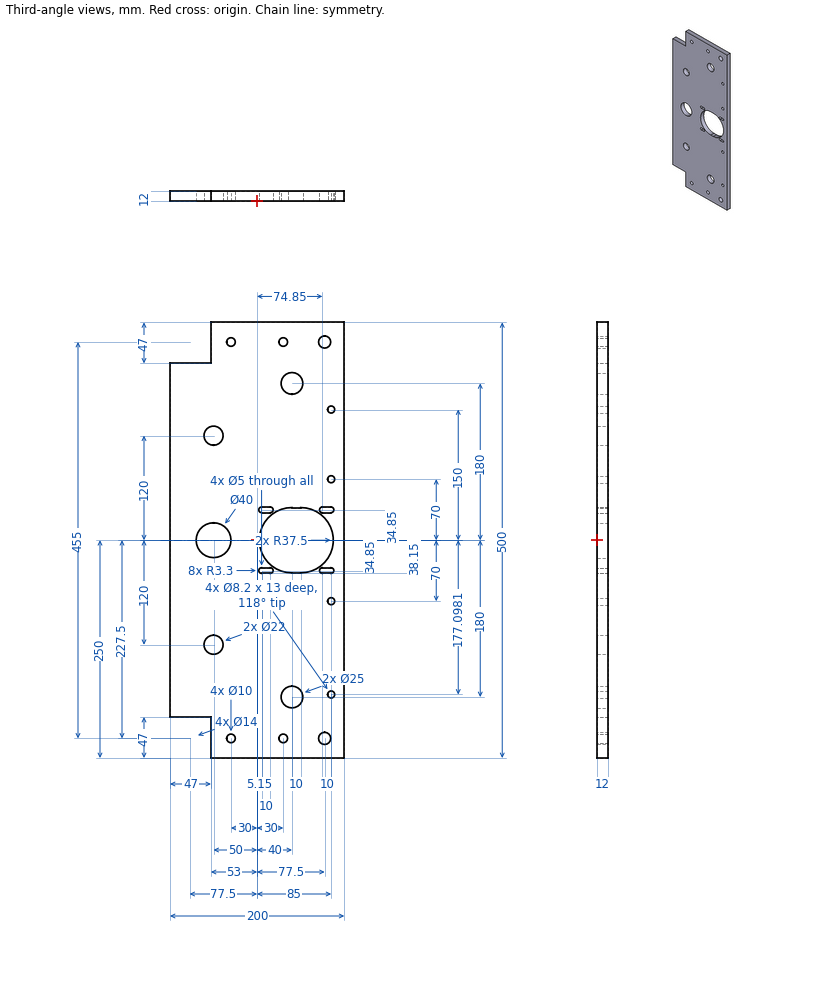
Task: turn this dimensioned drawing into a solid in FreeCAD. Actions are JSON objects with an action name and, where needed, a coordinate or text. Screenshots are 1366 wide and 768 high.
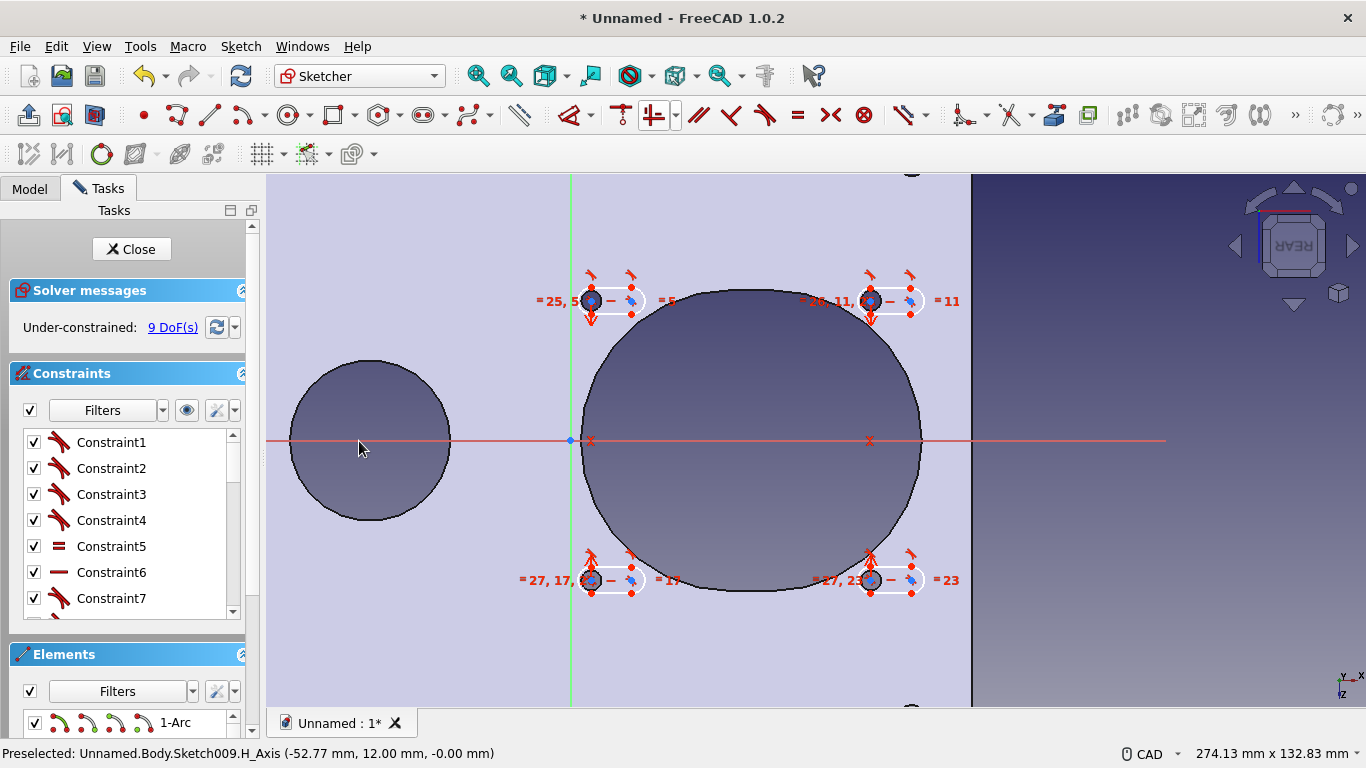
{"action": "scroll", "coordinate": [581, 293], "scroll_direction": "up", "scroll_amount": 6}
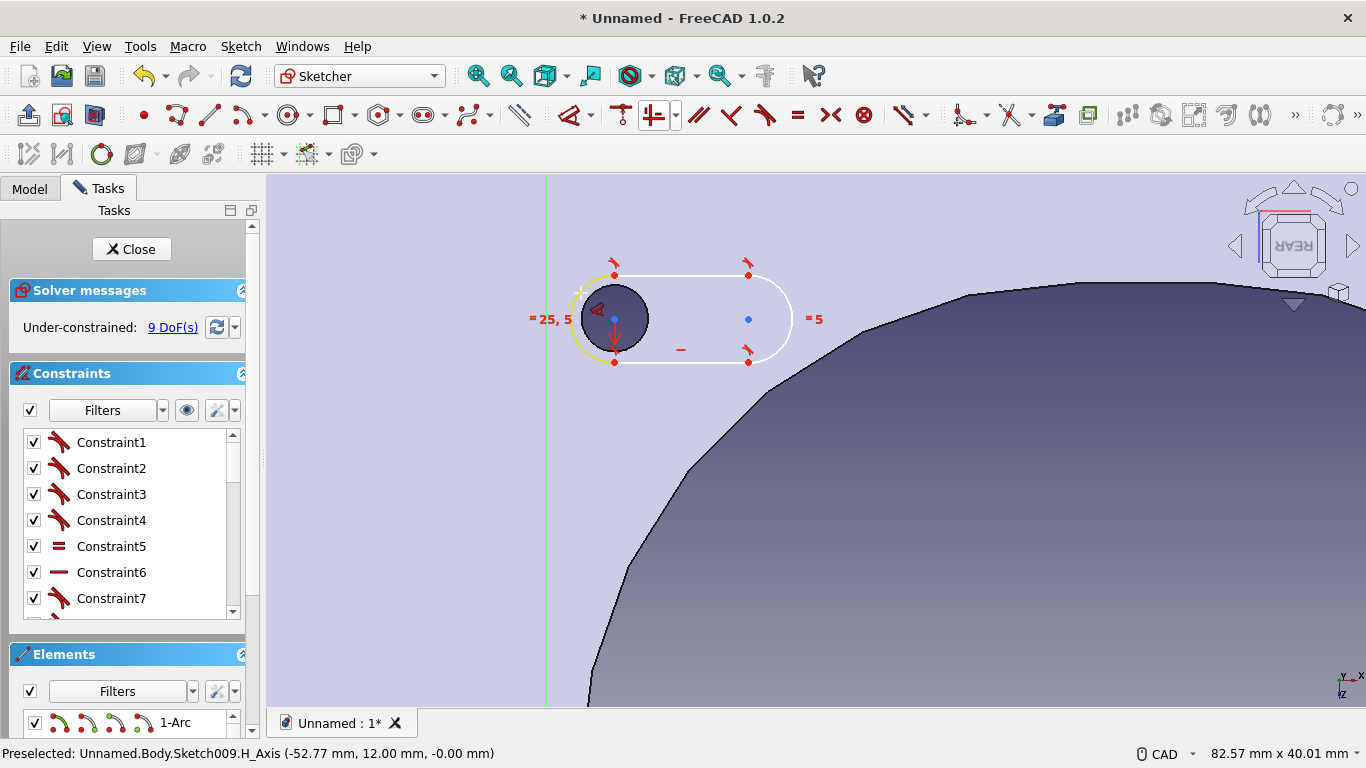
{"action": "left_click", "coordinate": [579, 294]}
{"action": "left_click", "coordinate": [581, 251]}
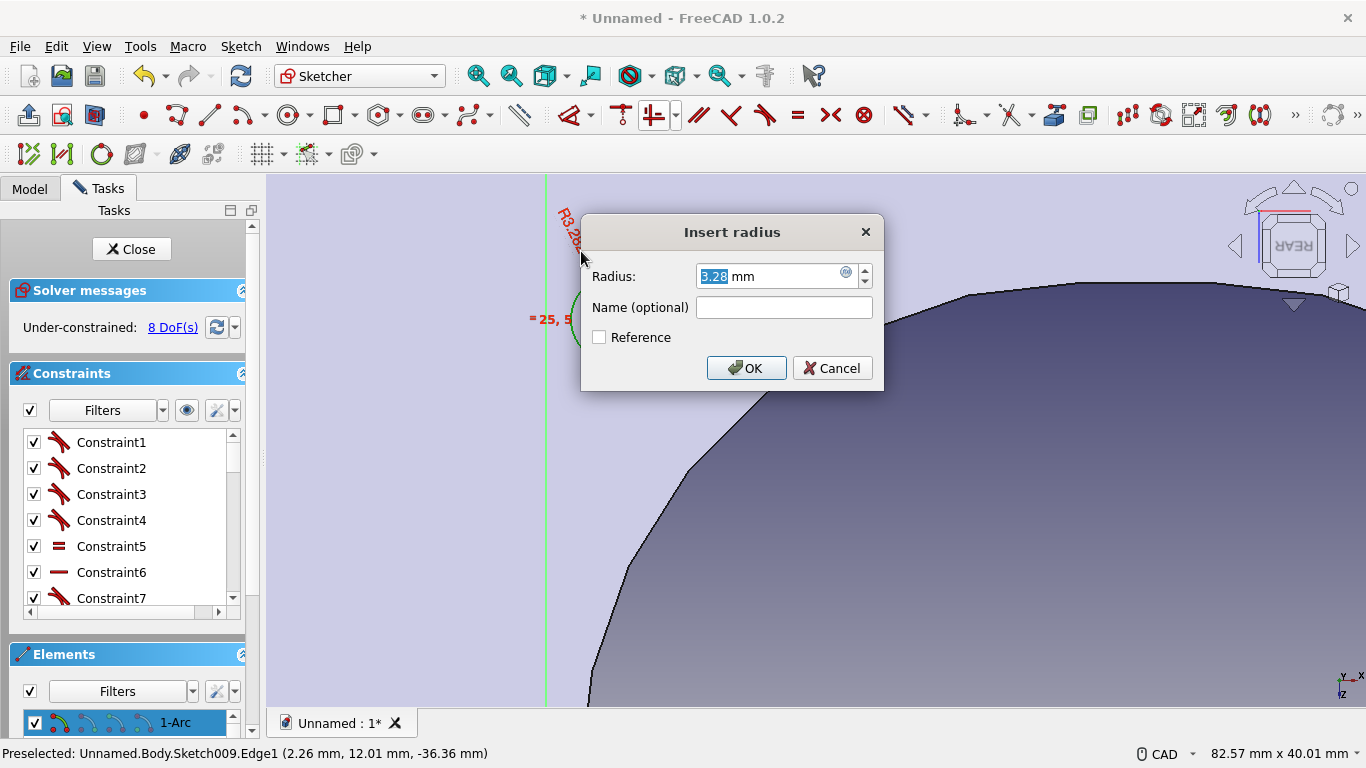
{"action": "type", "text": "3.3"}
{"action": "key", "text": "Return"}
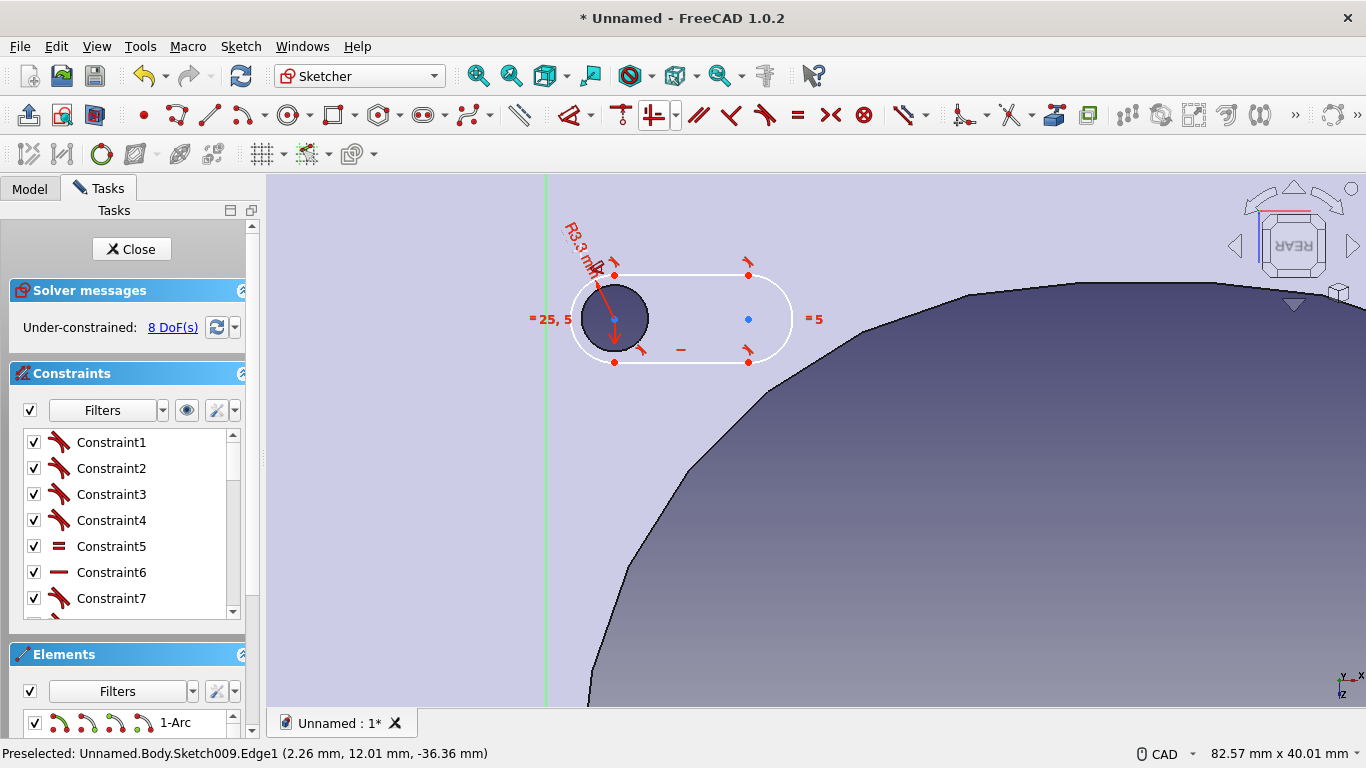
{"action": "left_click", "coordinate": [655, 275]}
{"action": "left_click", "coordinate": [682, 241]}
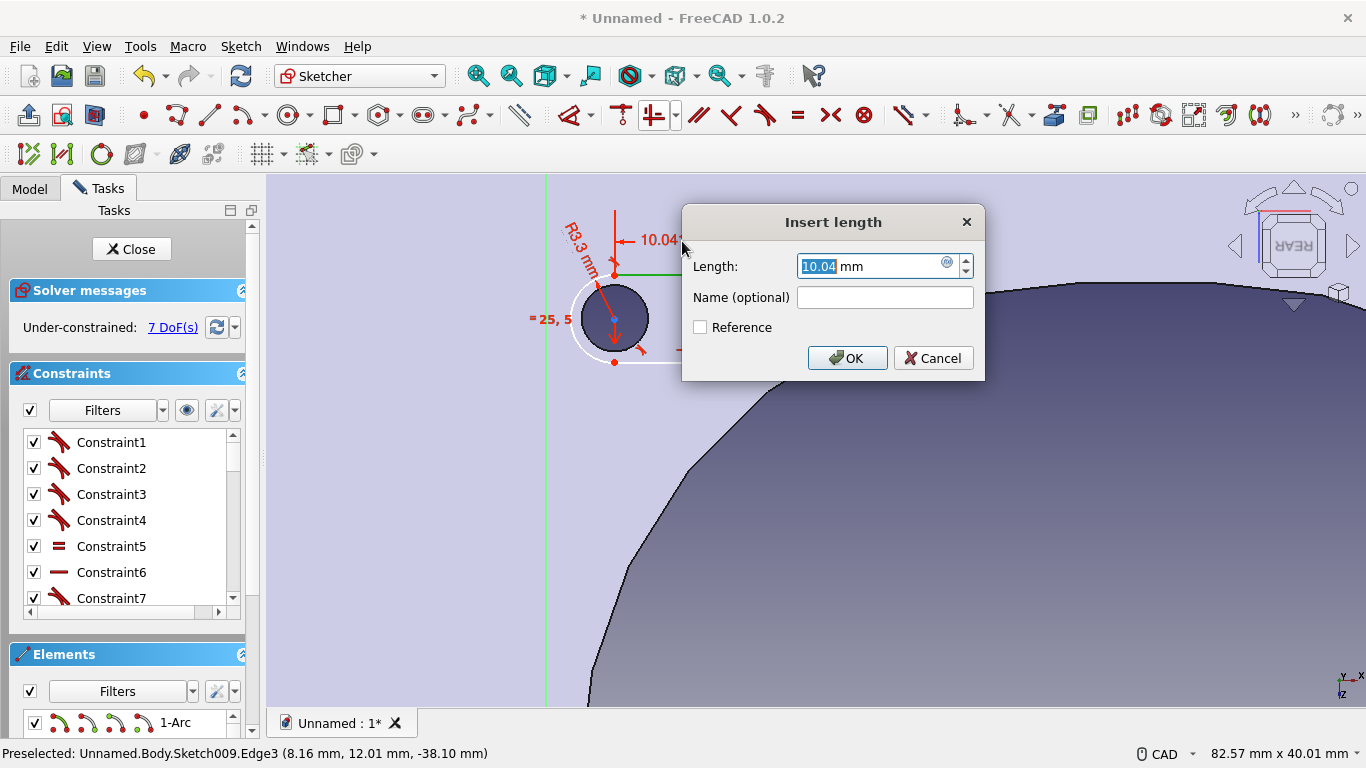
{"action": "type", "text": "10"}
{"action": "key", "text": "Return"}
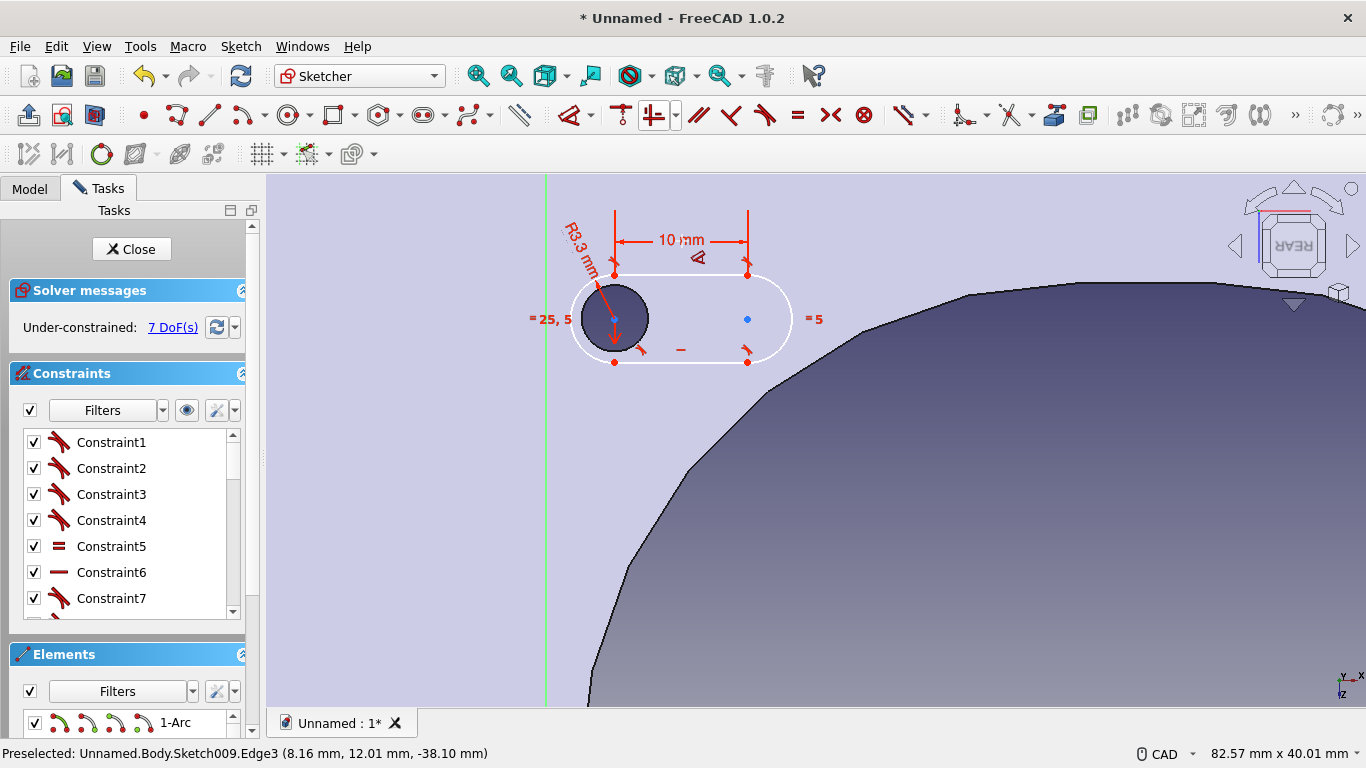
{"action": "scroll", "coordinate": [581, 293], "scroll_direction": "down", "scroll_amount": 6}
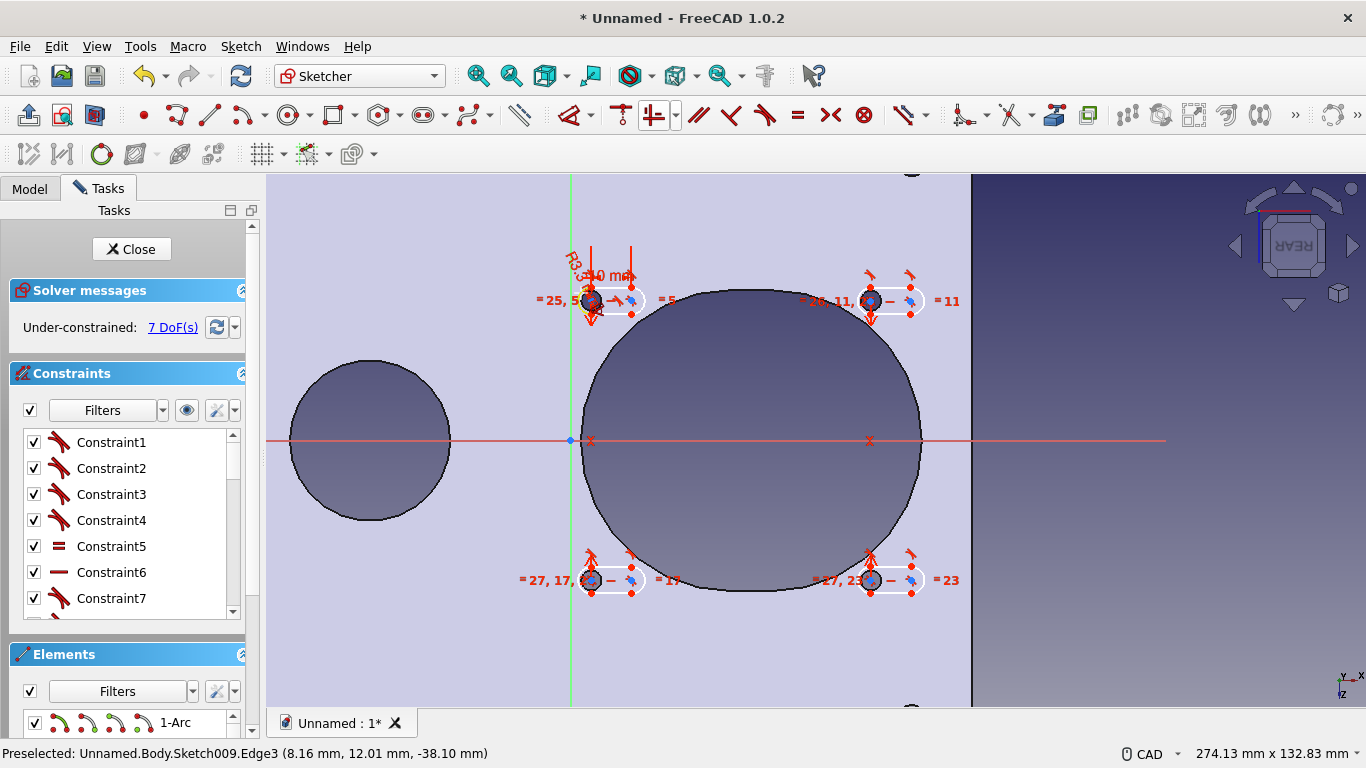
{"action": "left_click", "coordinate": [883, 288]}
{"action": "left_click", "coordinate": [891, 254]}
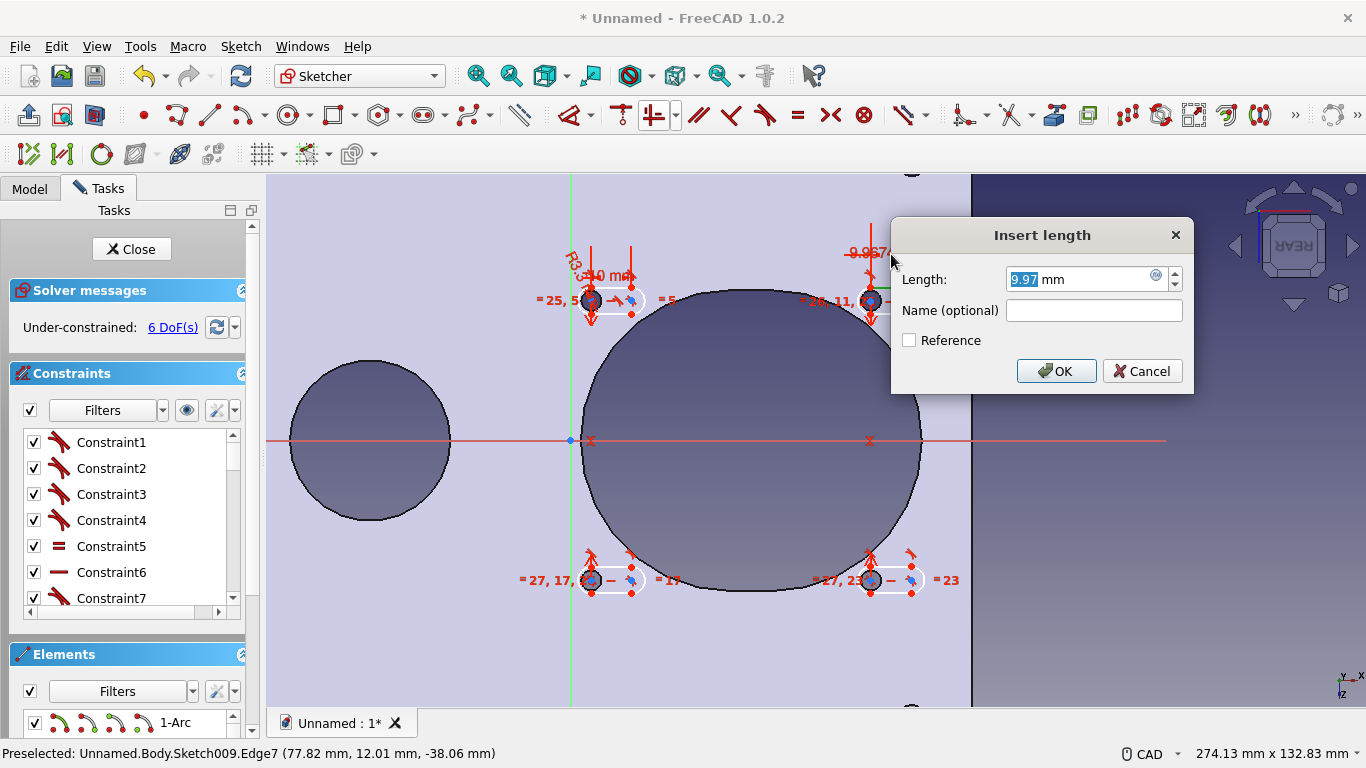
{"action": "type", "text": "10"}
{"action": "key", "text": "Return"}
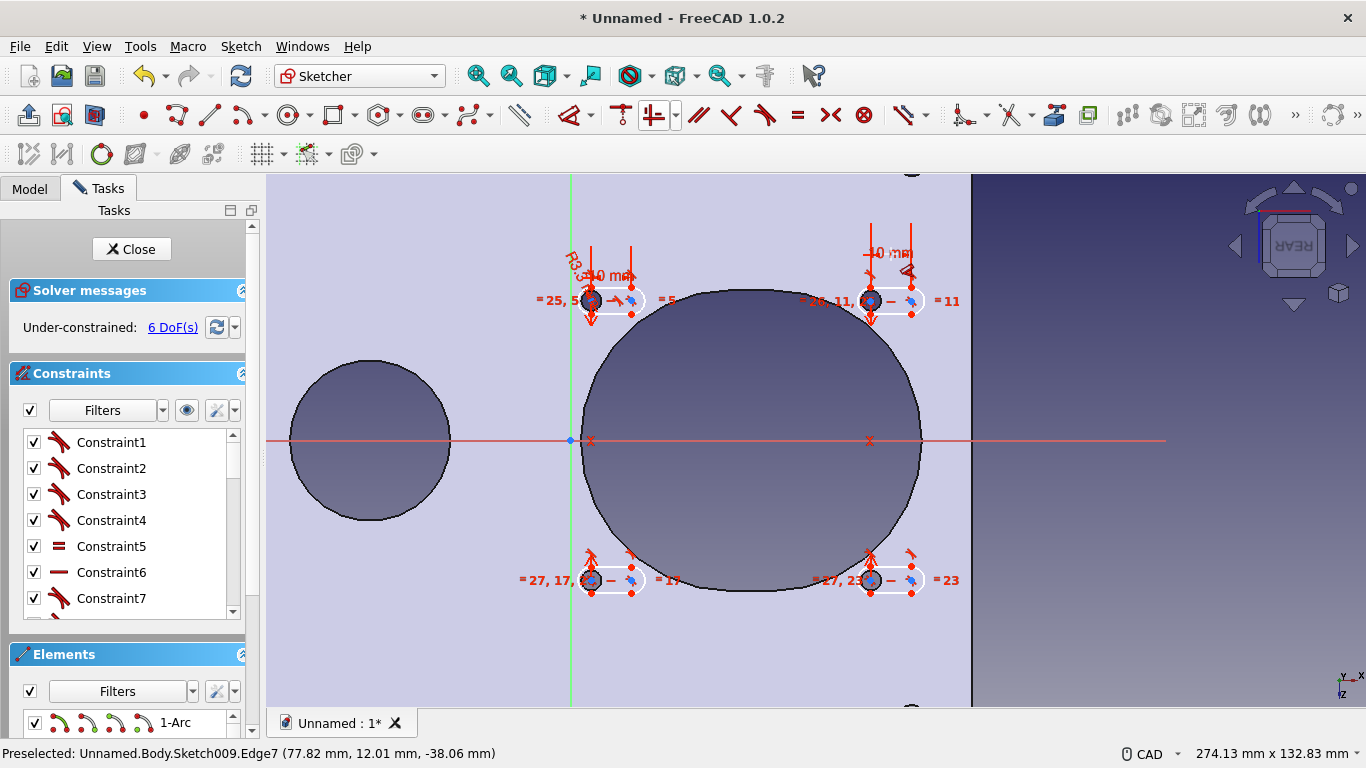
{"action": "left_click", "coordinate": [603, 567]}
{"action": "left_click", "coordinate": [612, 533]}